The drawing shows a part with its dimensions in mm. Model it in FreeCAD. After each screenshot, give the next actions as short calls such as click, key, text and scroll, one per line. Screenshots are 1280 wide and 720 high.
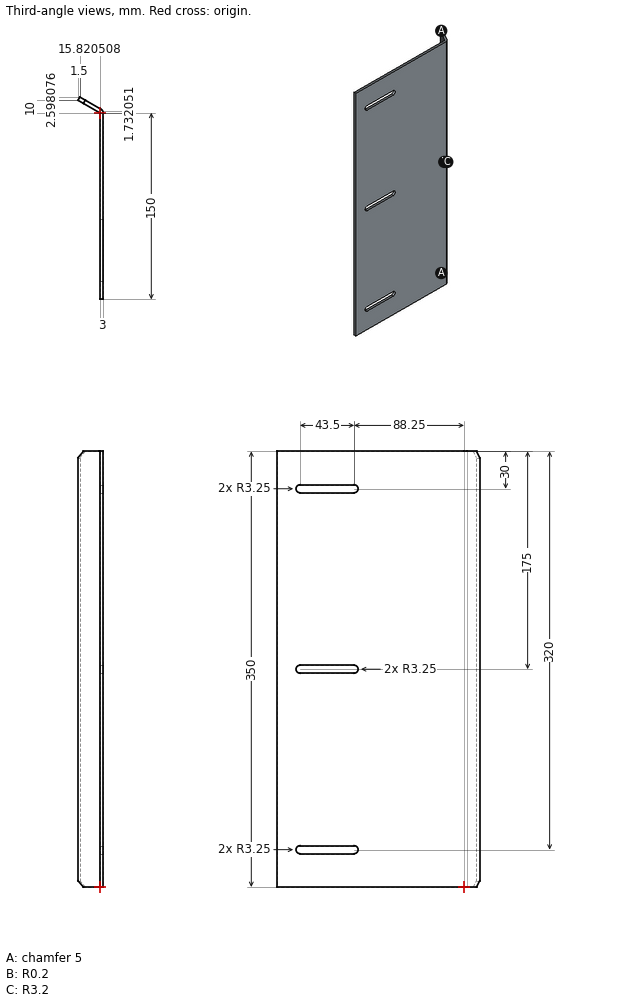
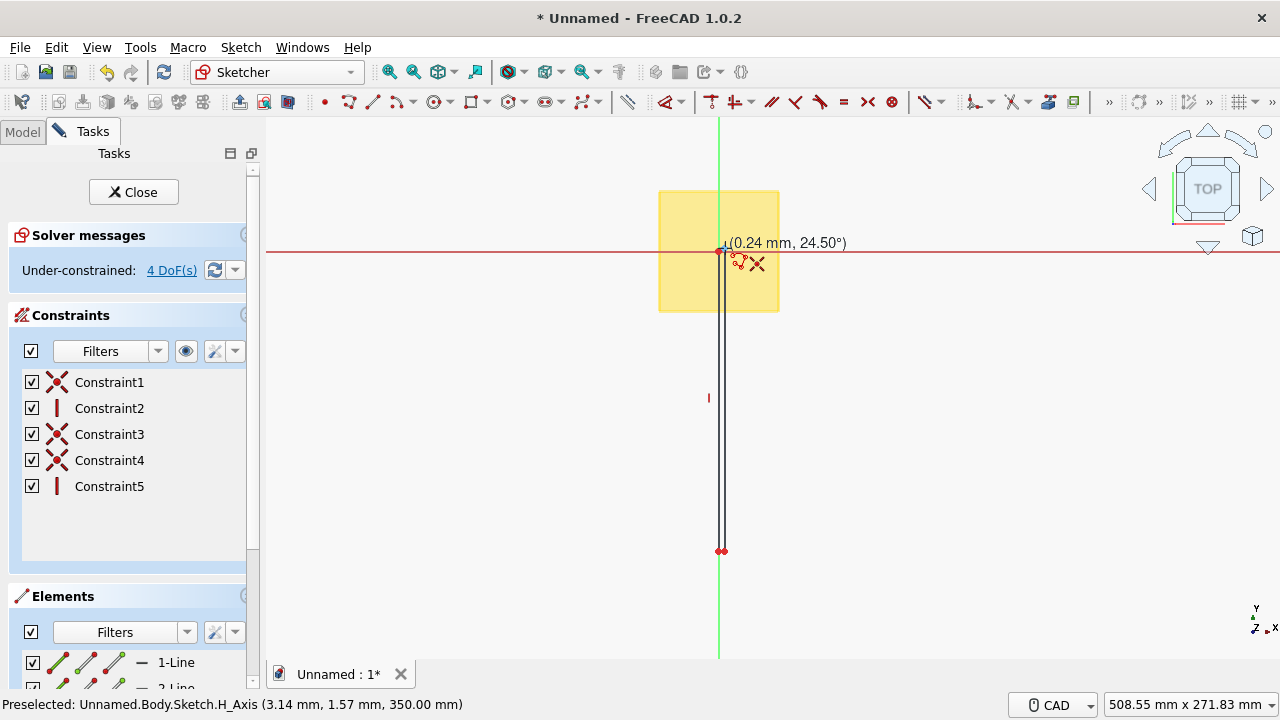
click(687, 226)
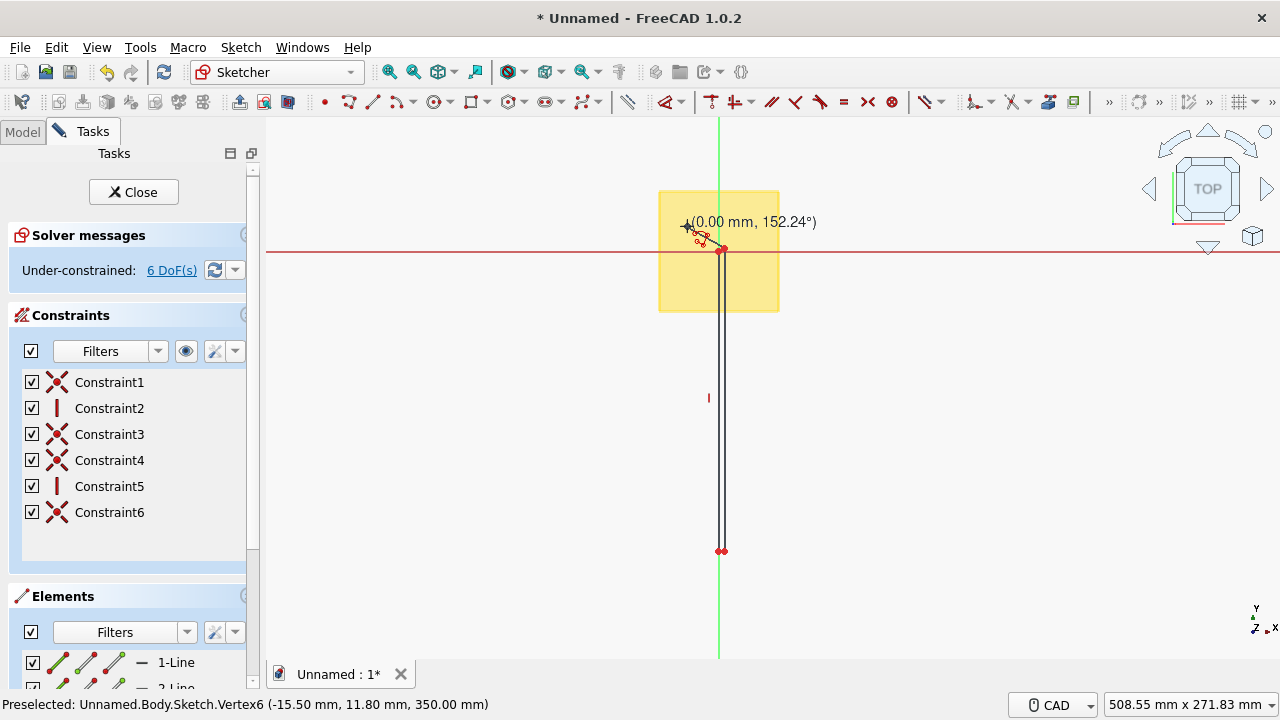
scroll(684, 232, up, 5)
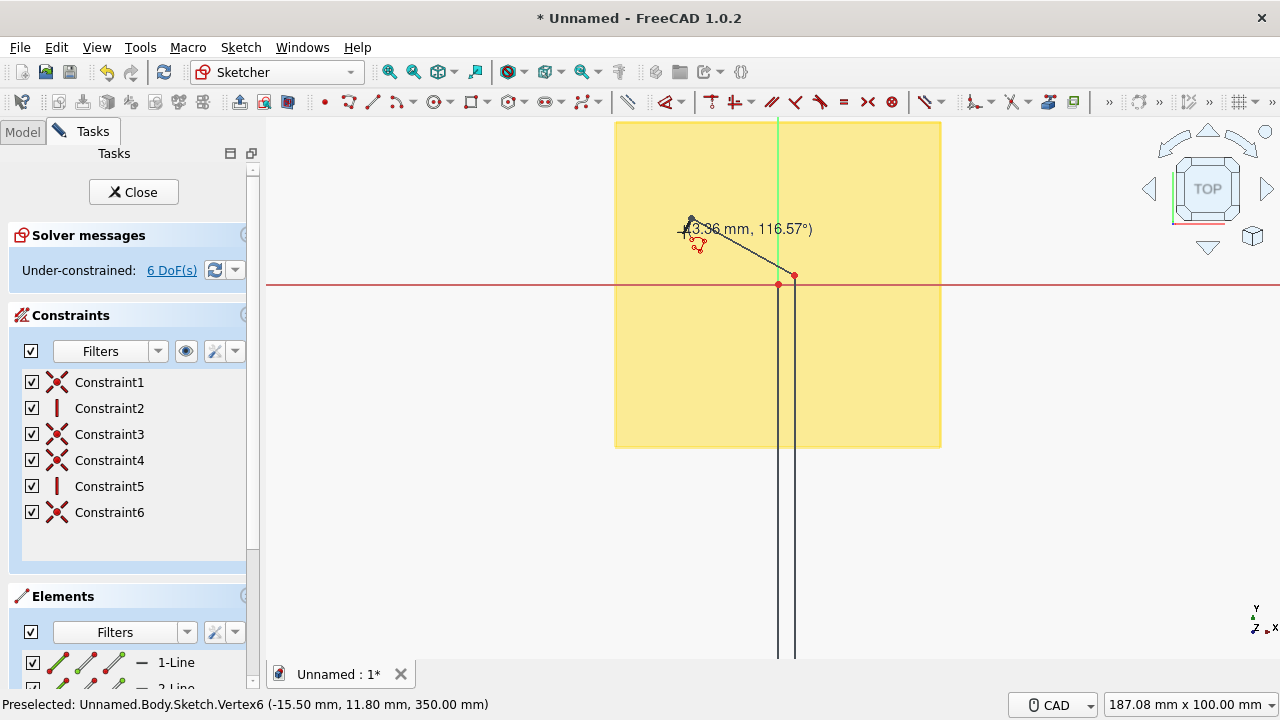
click(684, 231)
click(778, 285)
key(Escape)
key(Escape)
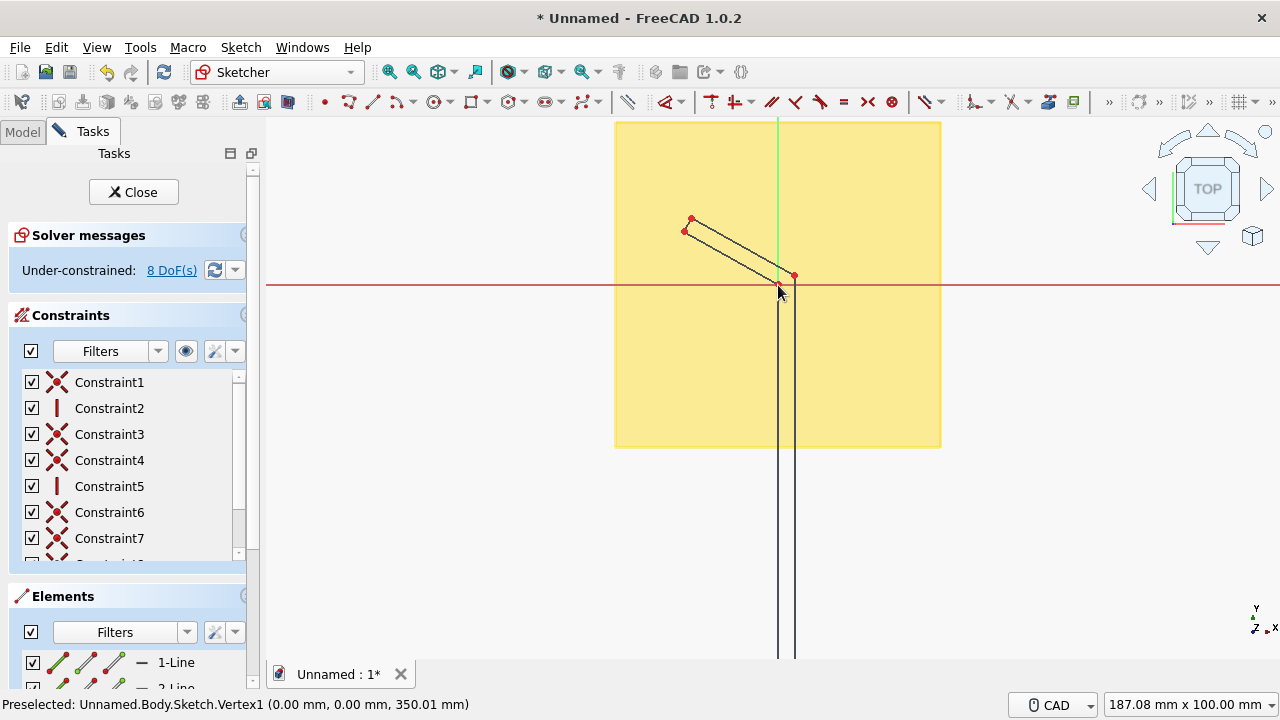
scroll(684, 231, down, 5)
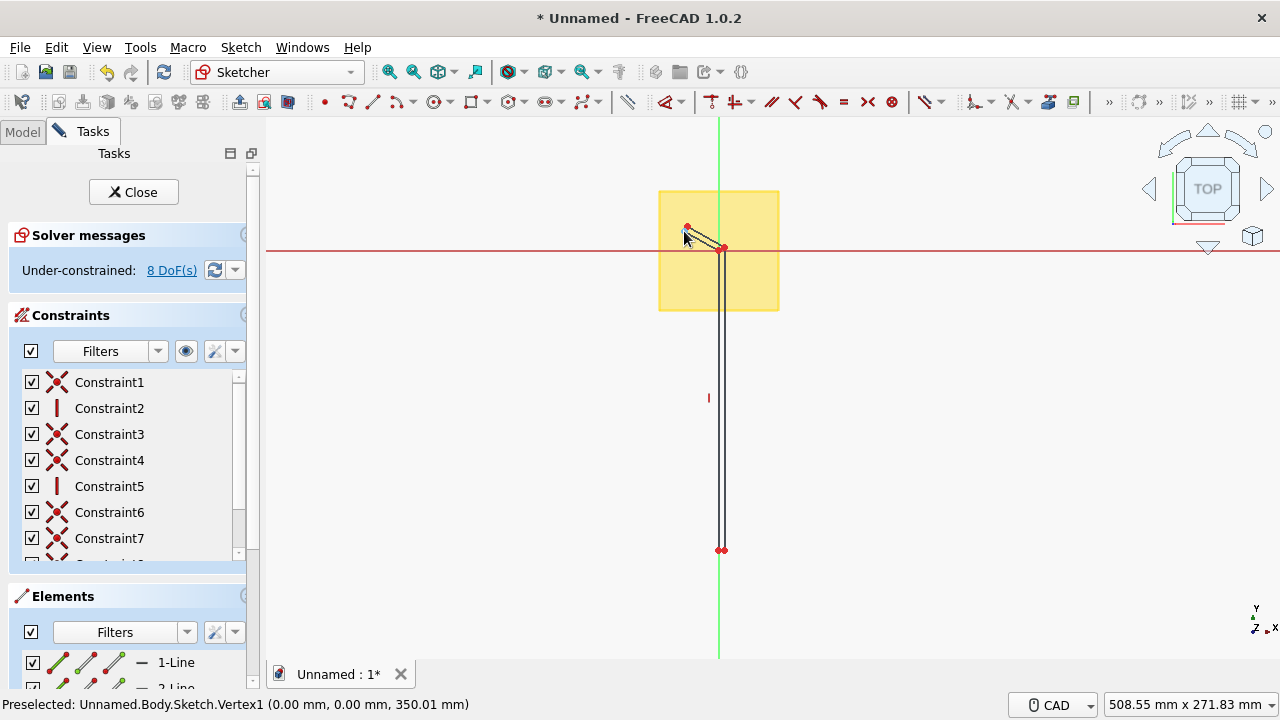
scroll(722, 551, up, 8)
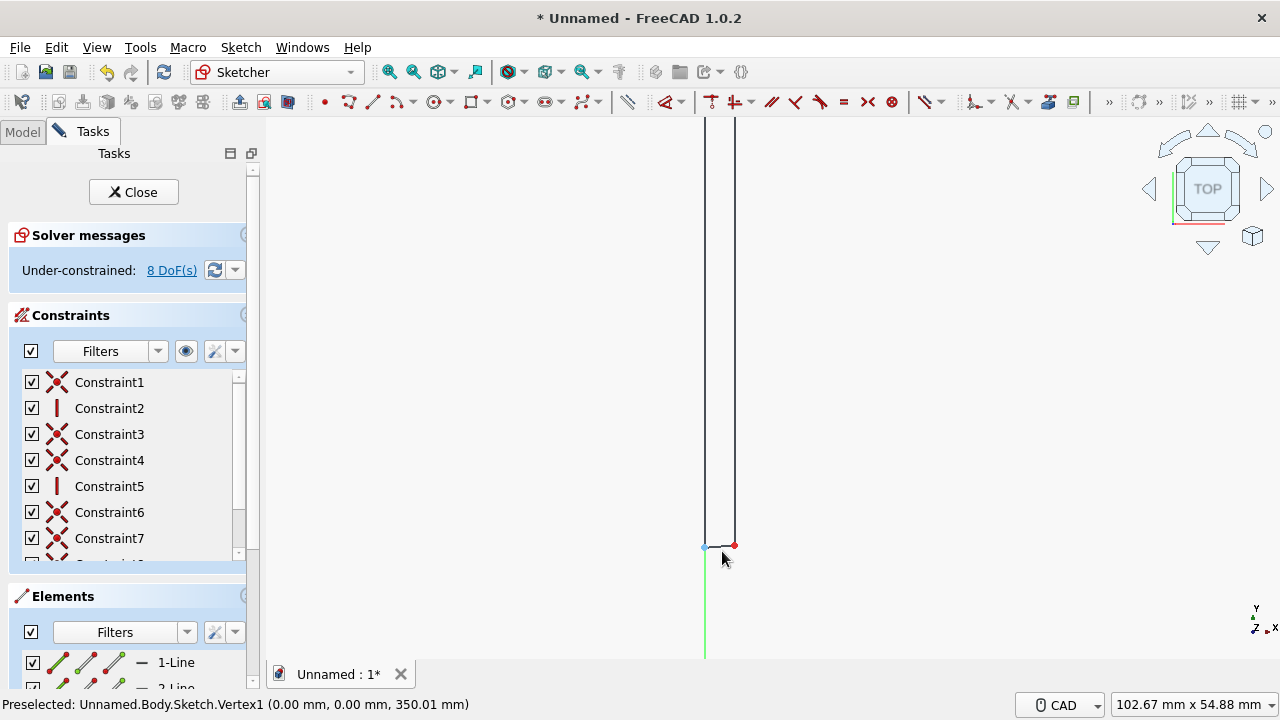
click(720, 547)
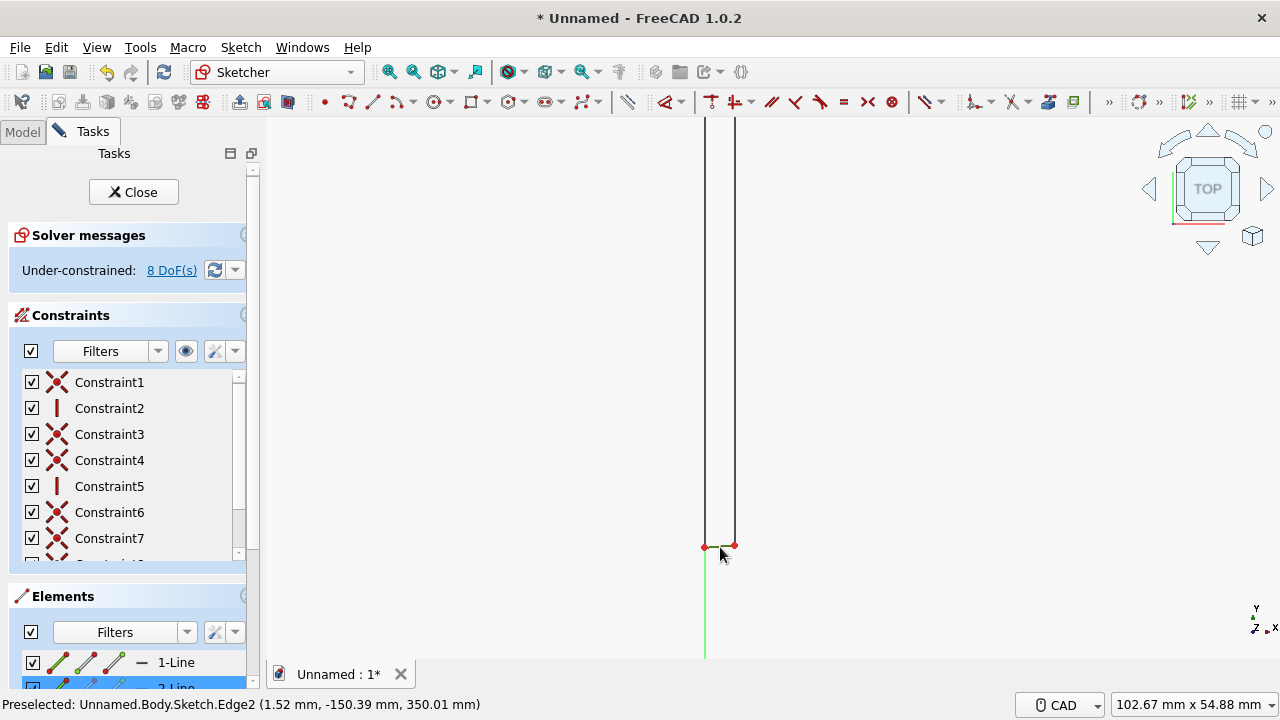
key(h)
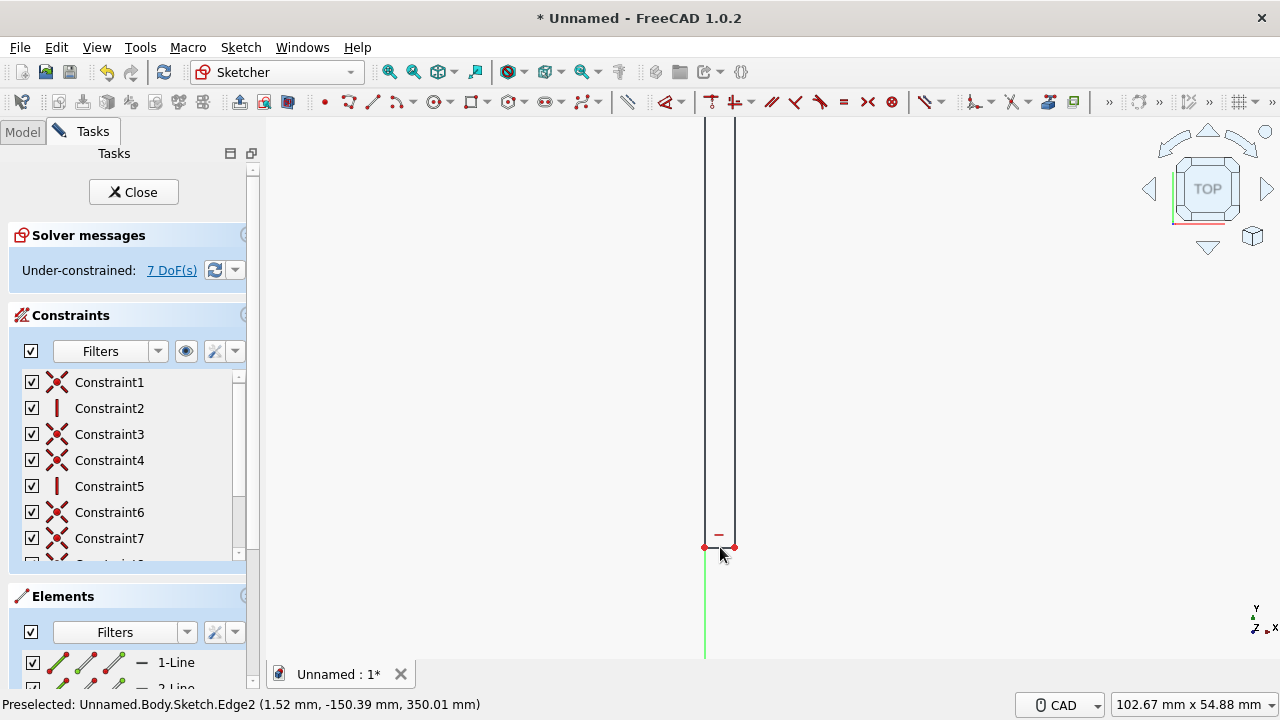
key(d)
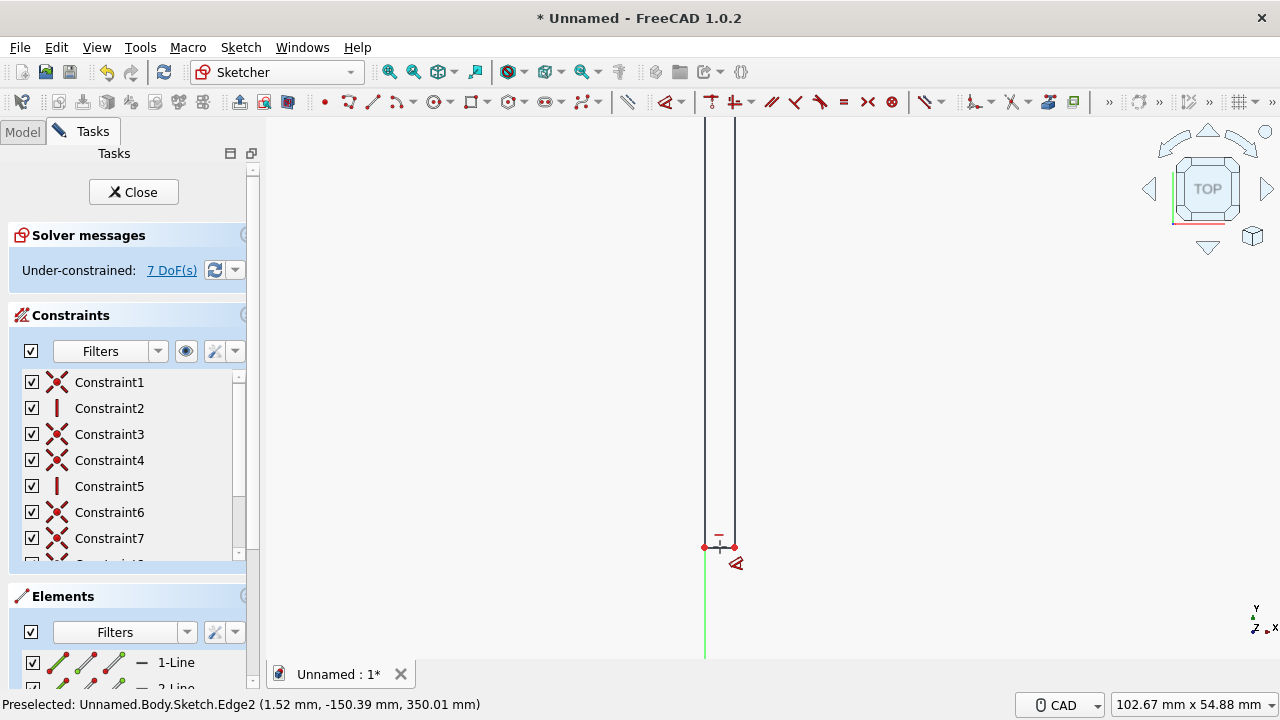
scroll(717, 548, up, 2)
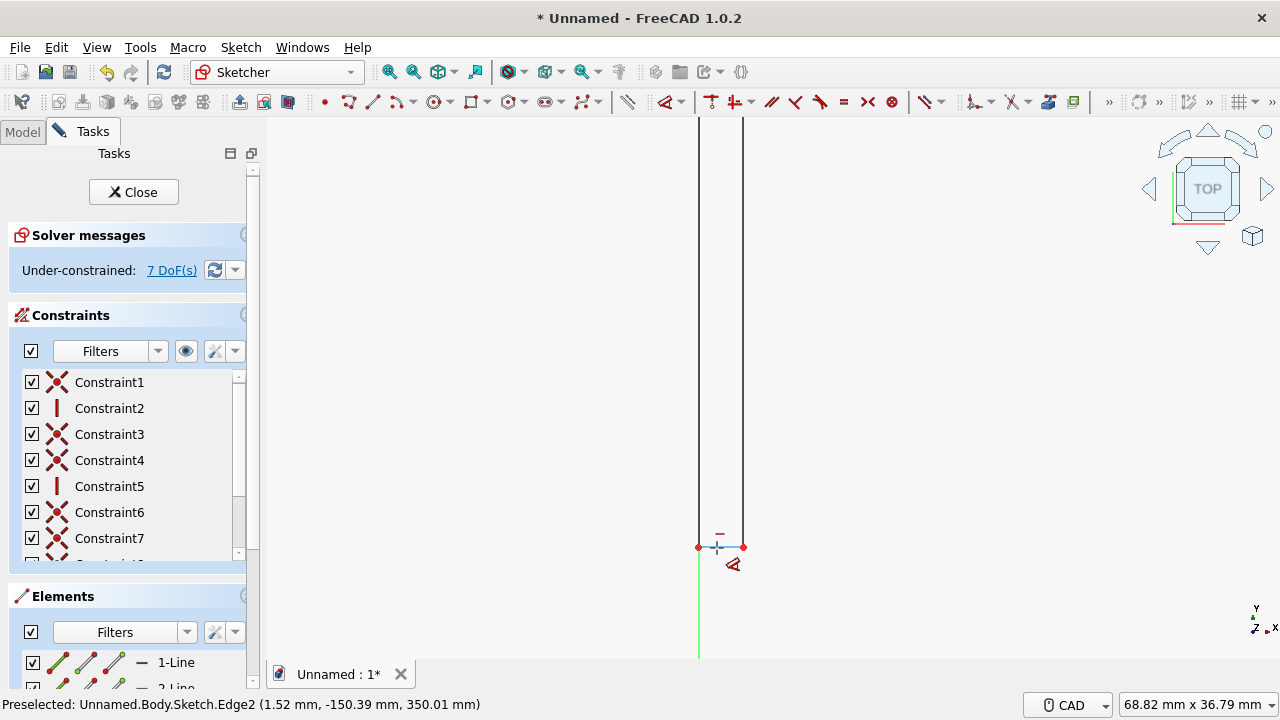
click(716, 547)
click(721, 581)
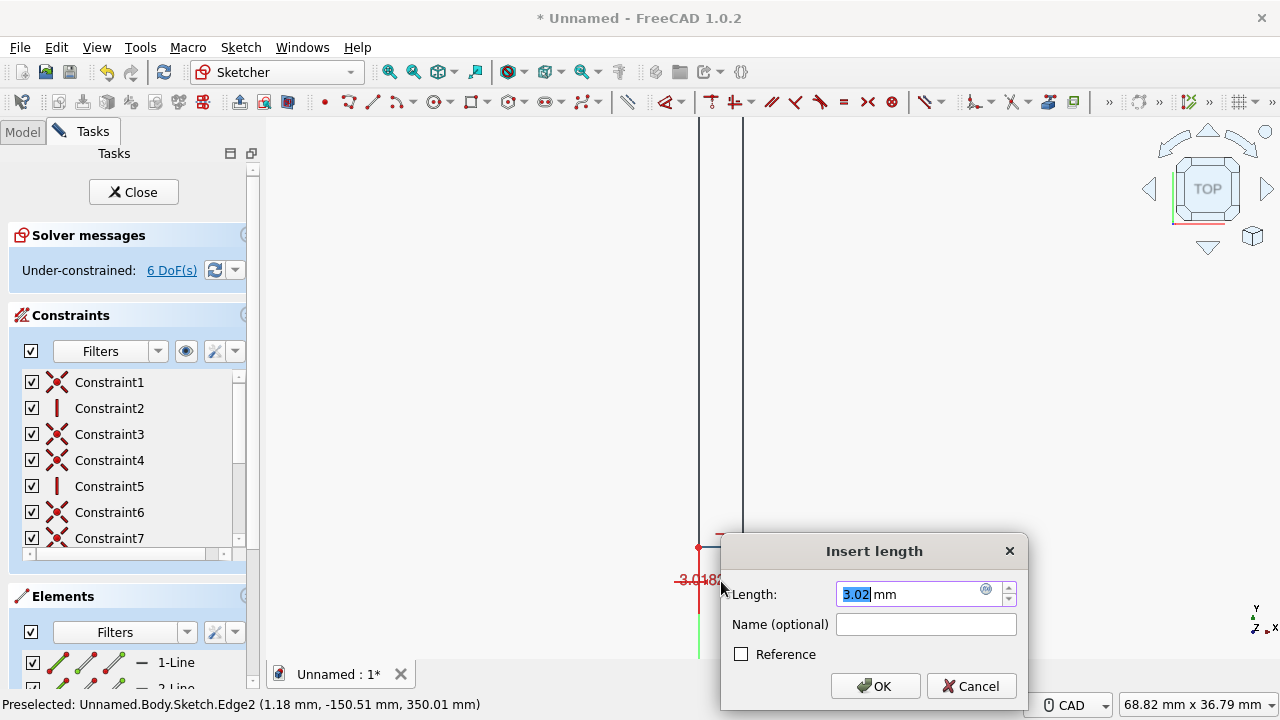
text(3)
key(Return)